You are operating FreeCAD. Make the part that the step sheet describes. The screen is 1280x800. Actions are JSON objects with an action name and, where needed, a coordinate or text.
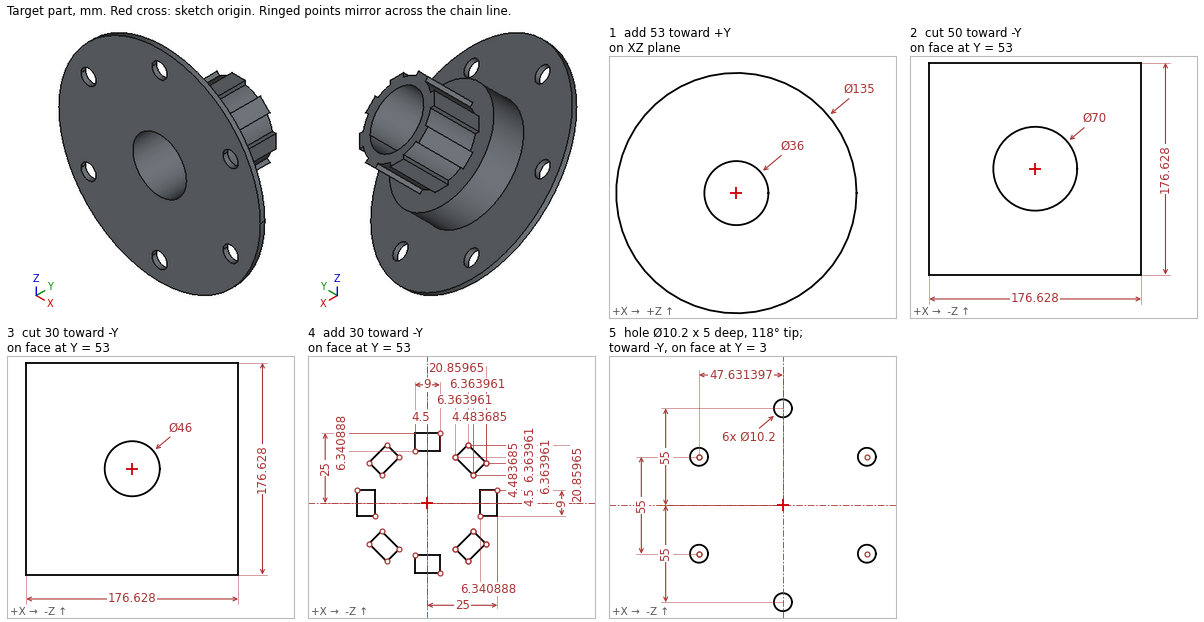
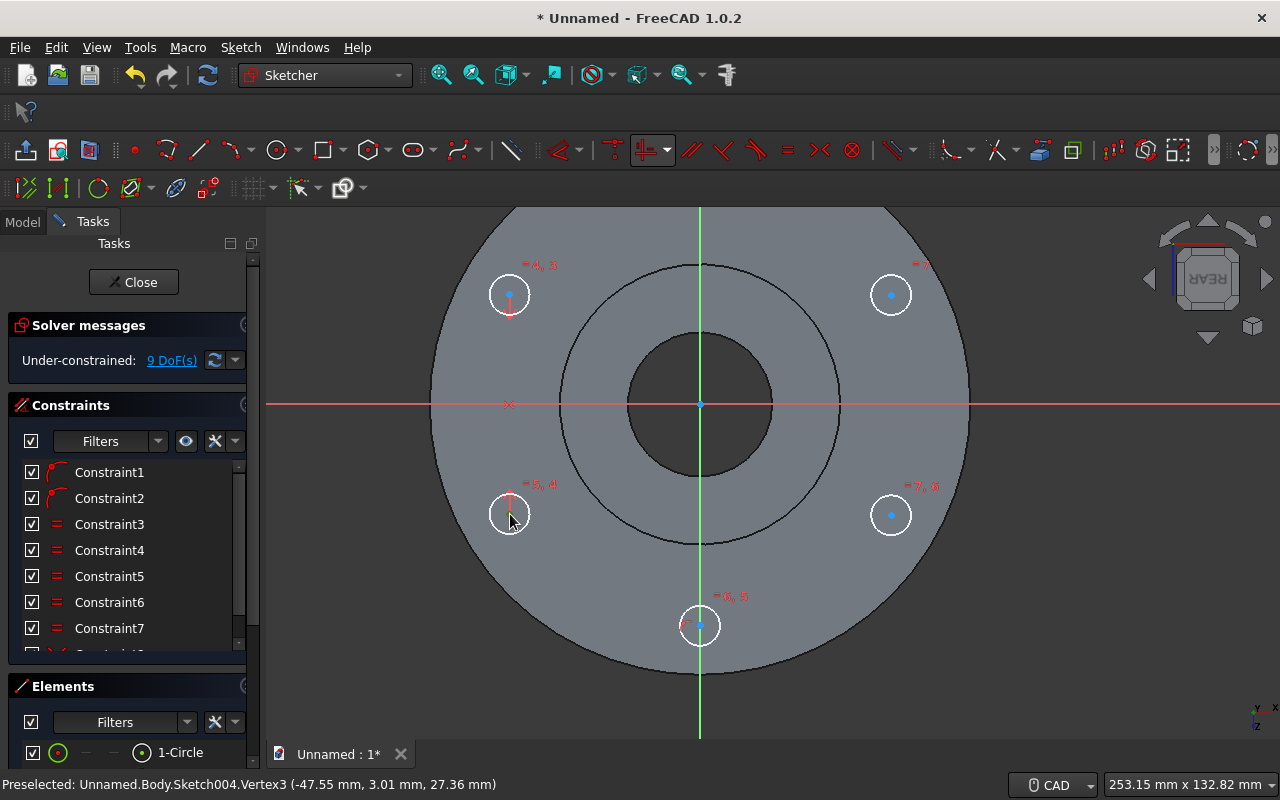
{"action": "left_click", "coordinate": [891, 515]}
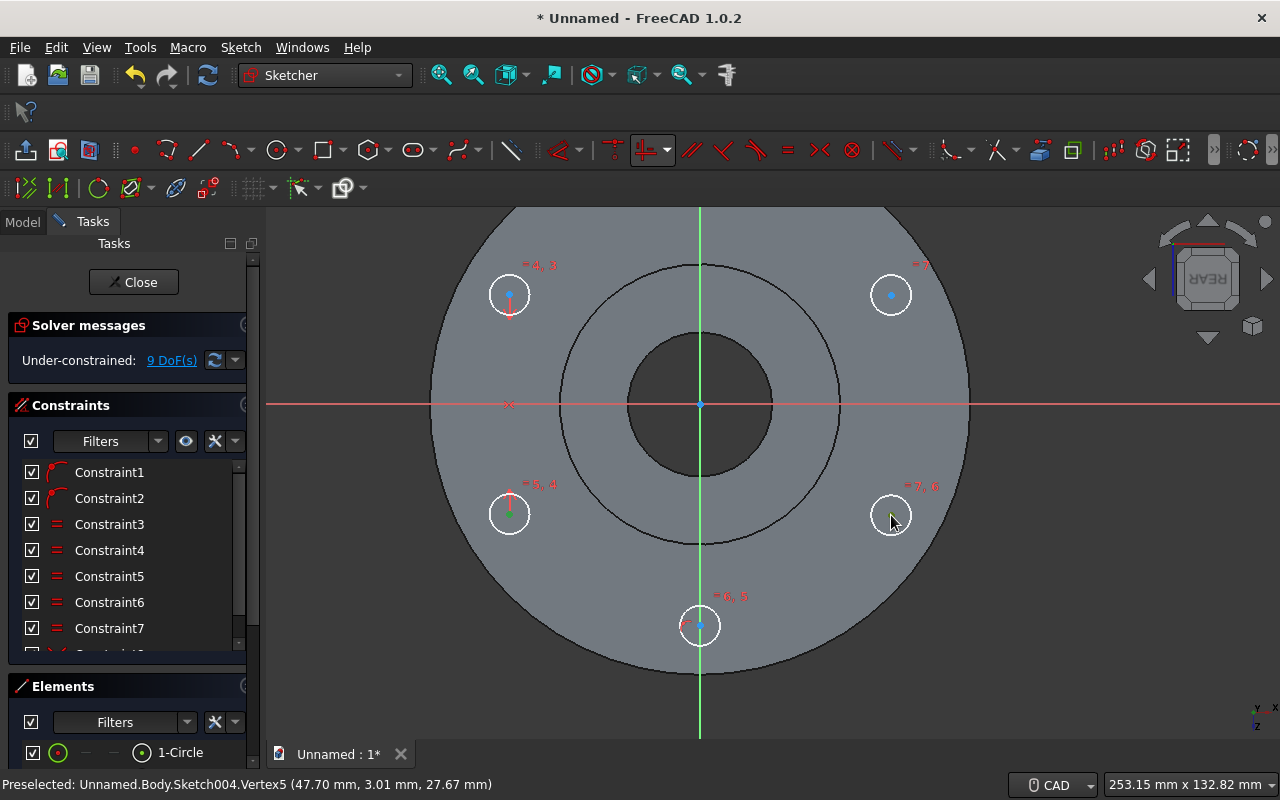
{"action": "left_click", "coordinate": [700, 677]}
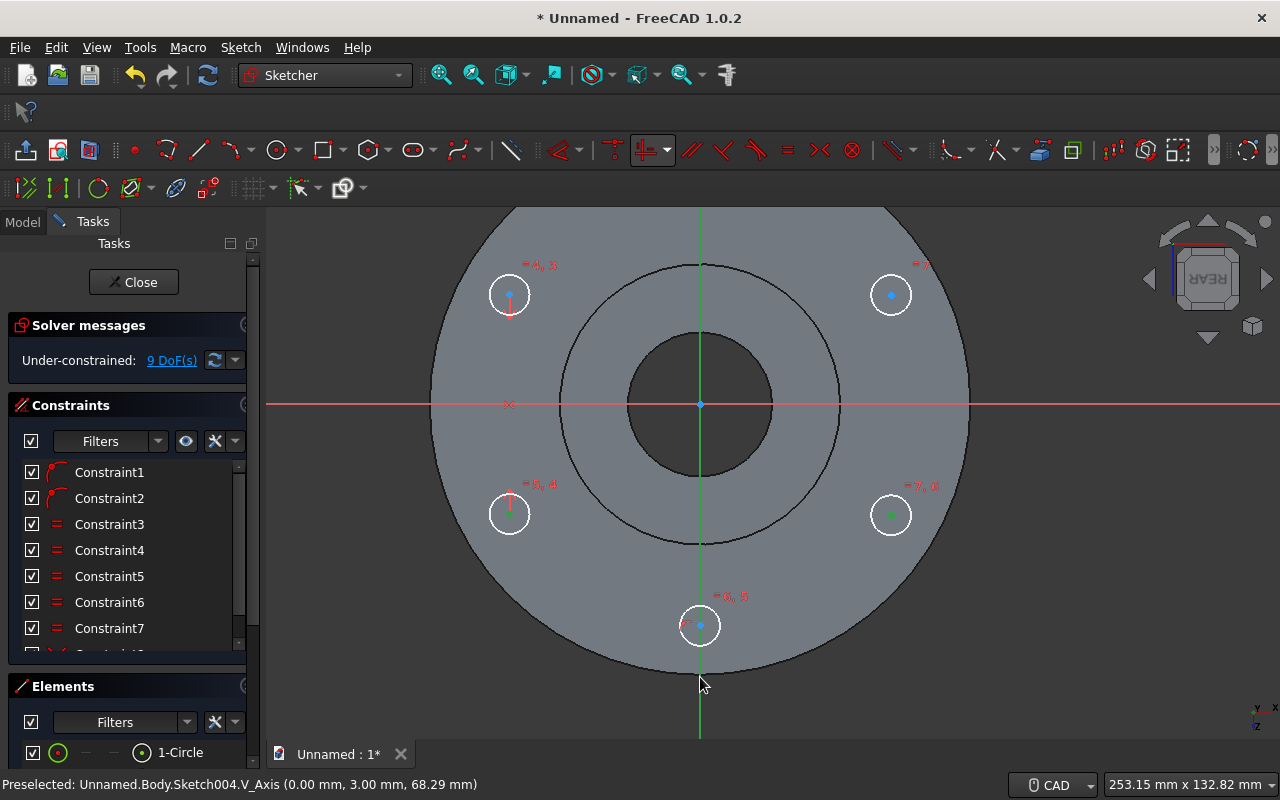
{"action": "left_click", "coordinate": [820, 150]}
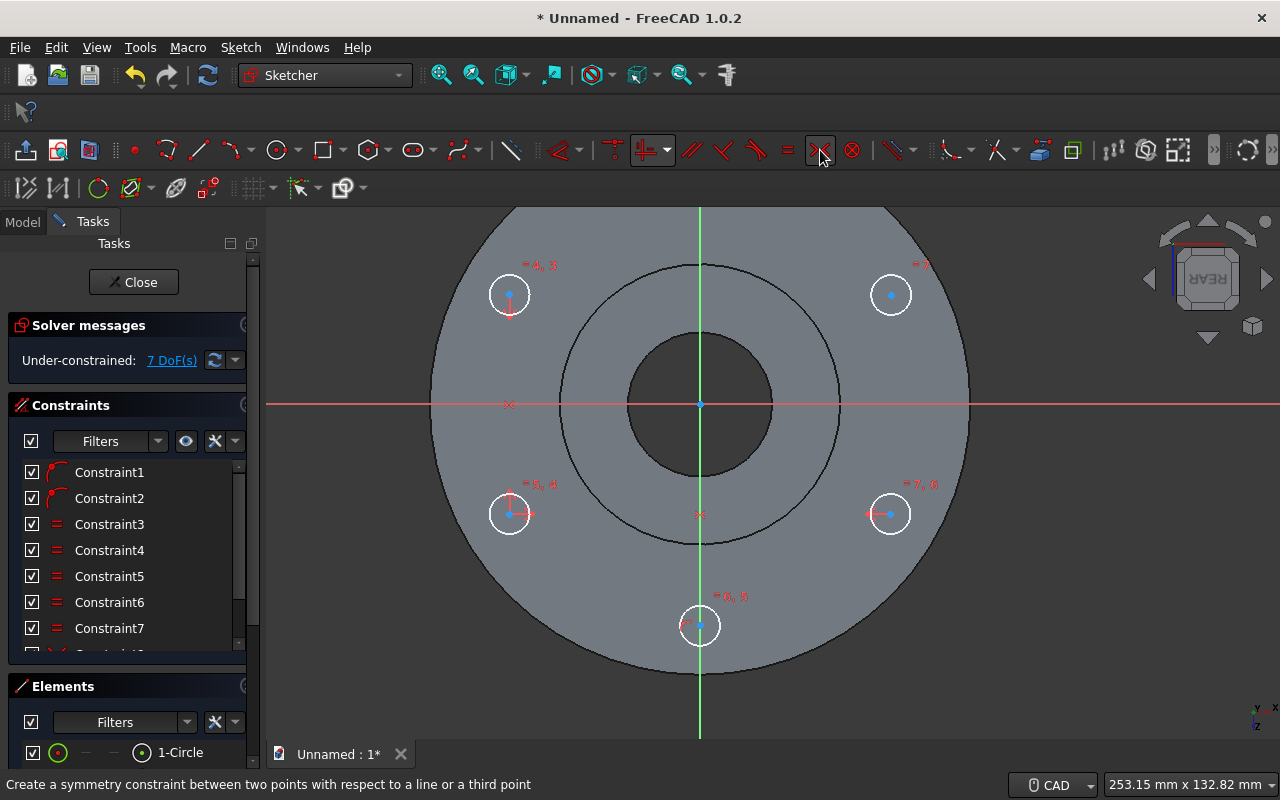
{"action": "left_click", "coordinate": [510, 295]}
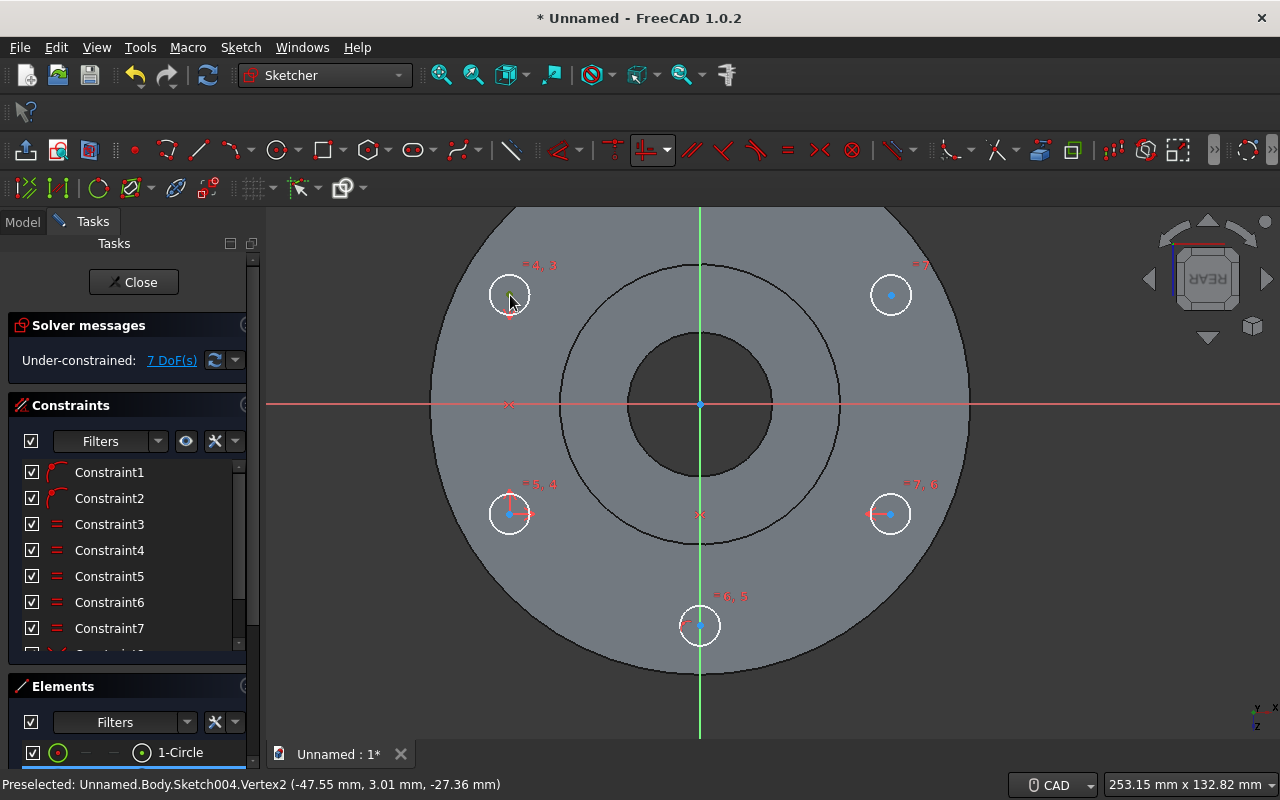
{"action": "left_click", "coordinate": [891, 295]}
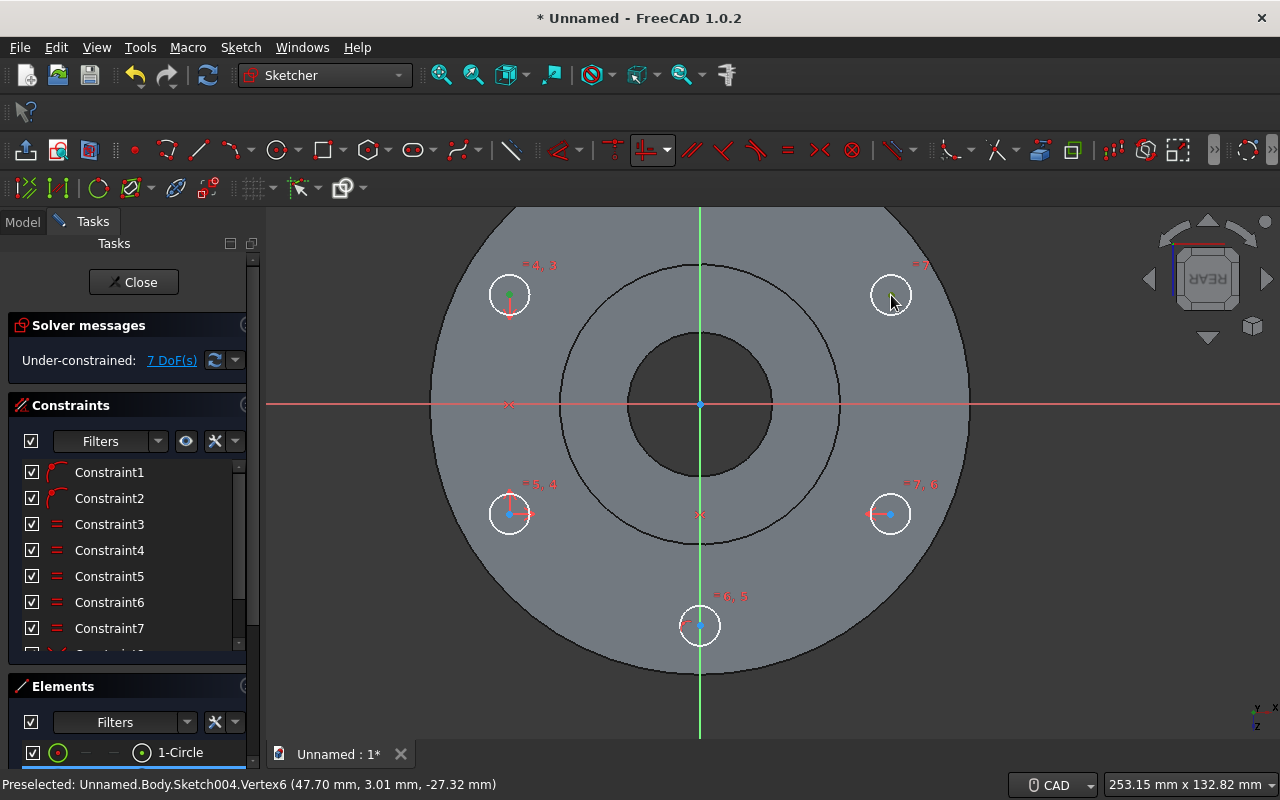
{"action": "left_click", "coordinate": [700, 677]}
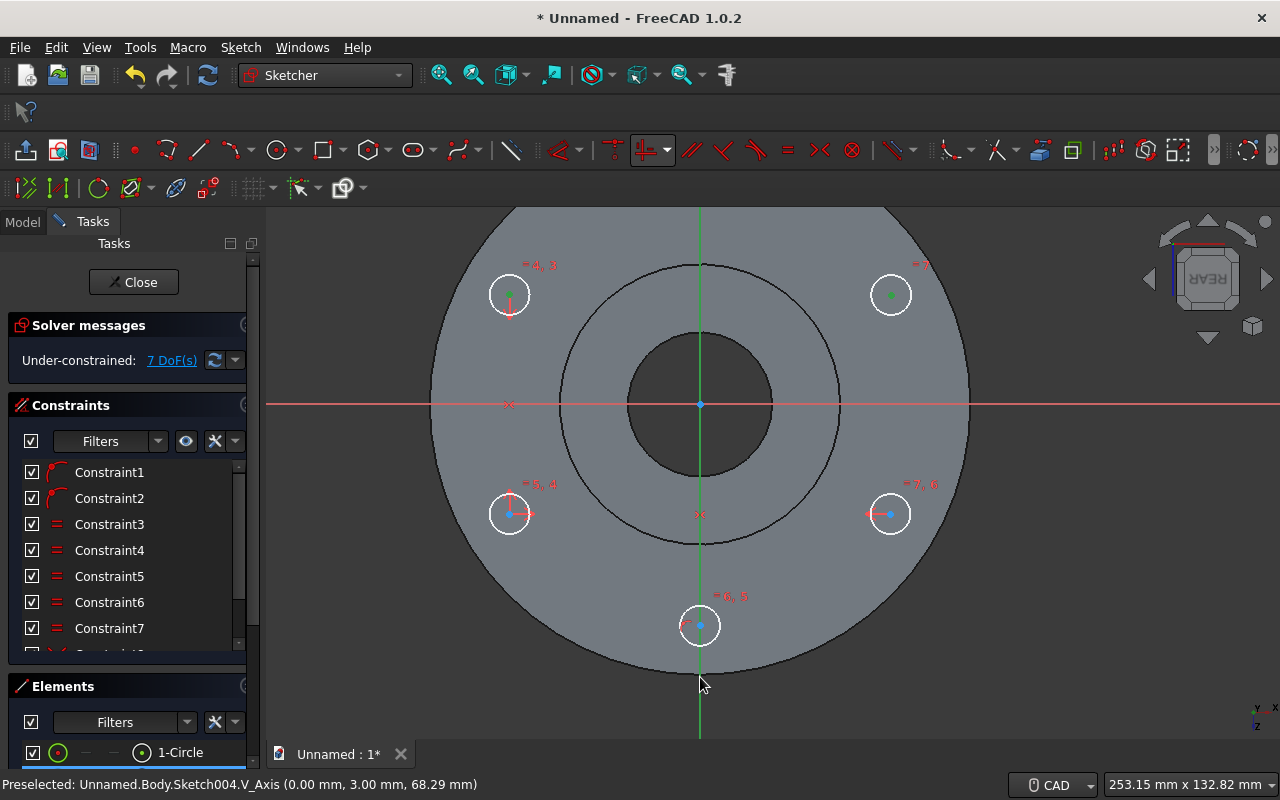
{"action": "left_click", "coordinate": [820, 150]}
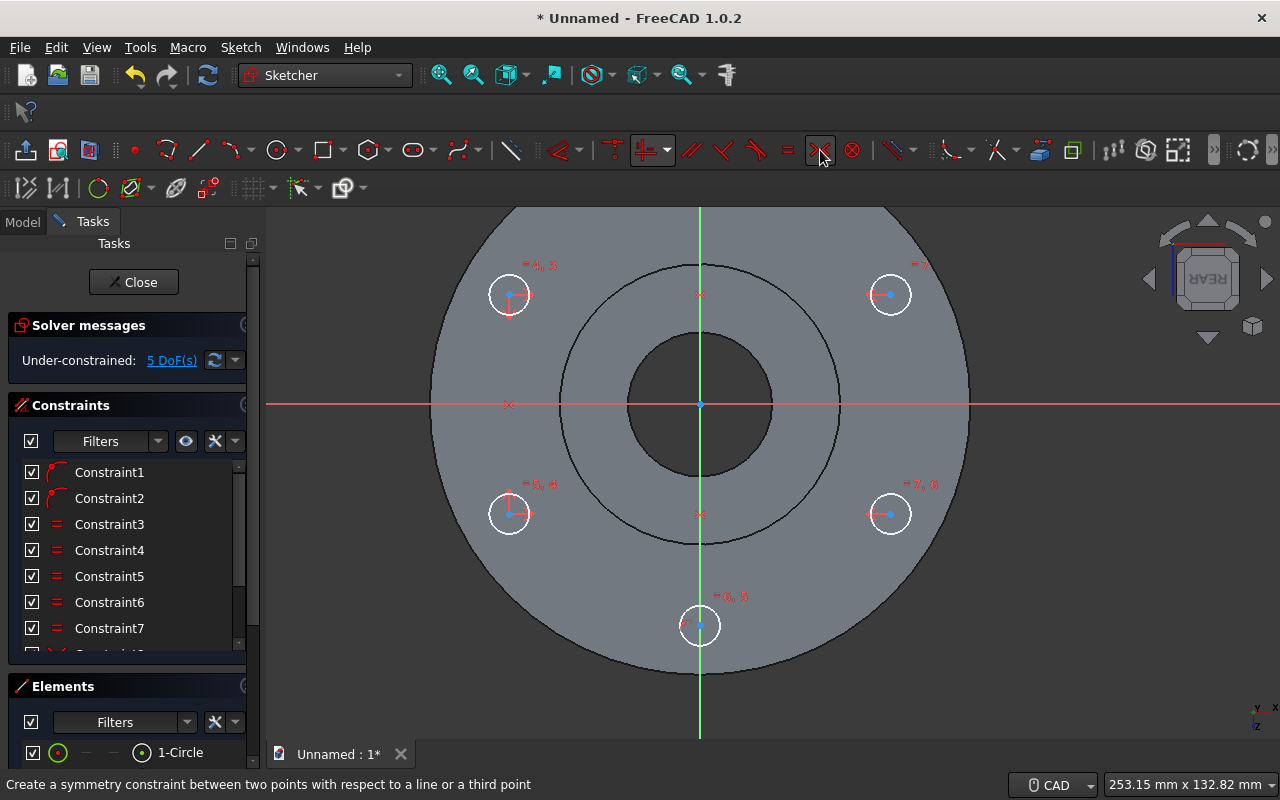
{"action": "left_click", "coordinate": [558, 150]}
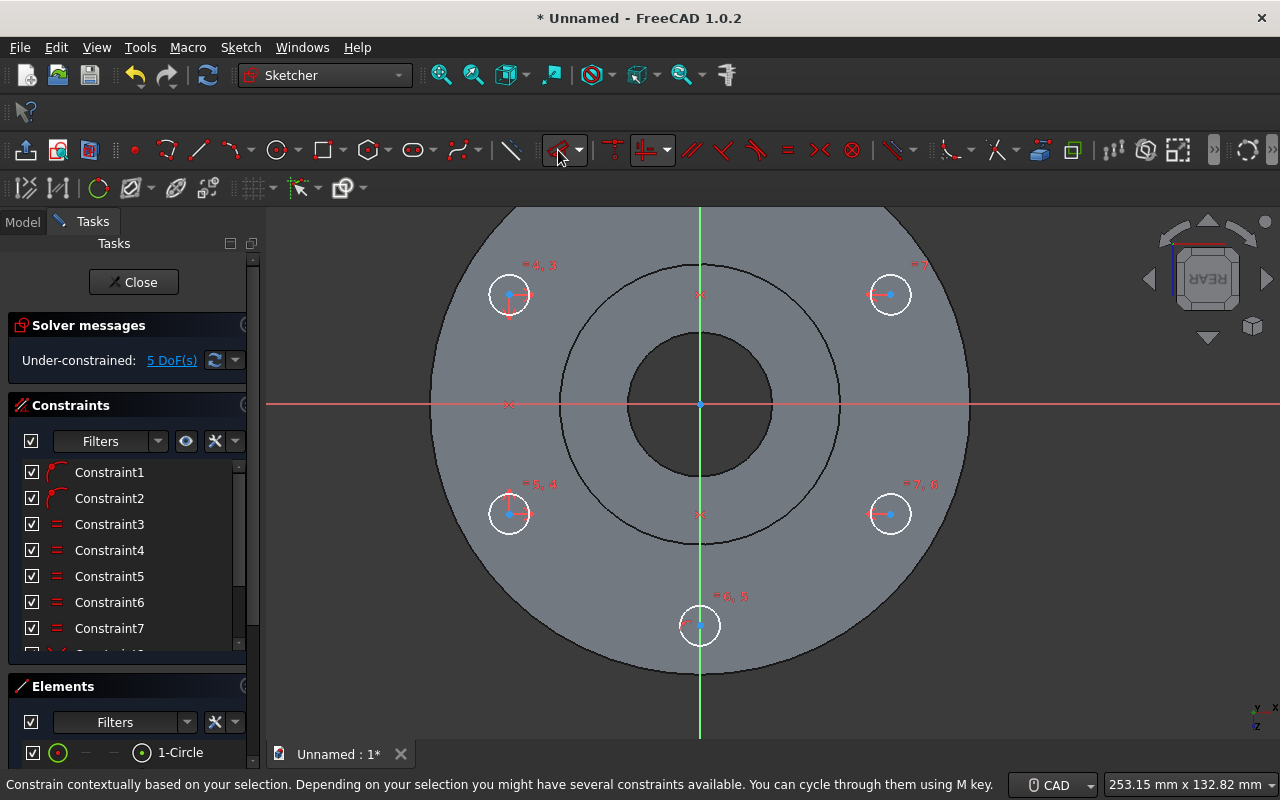
{"action": "scroll", "coordinate": [714, 612], "scroll_direction": "down", "scroll_amount": 2}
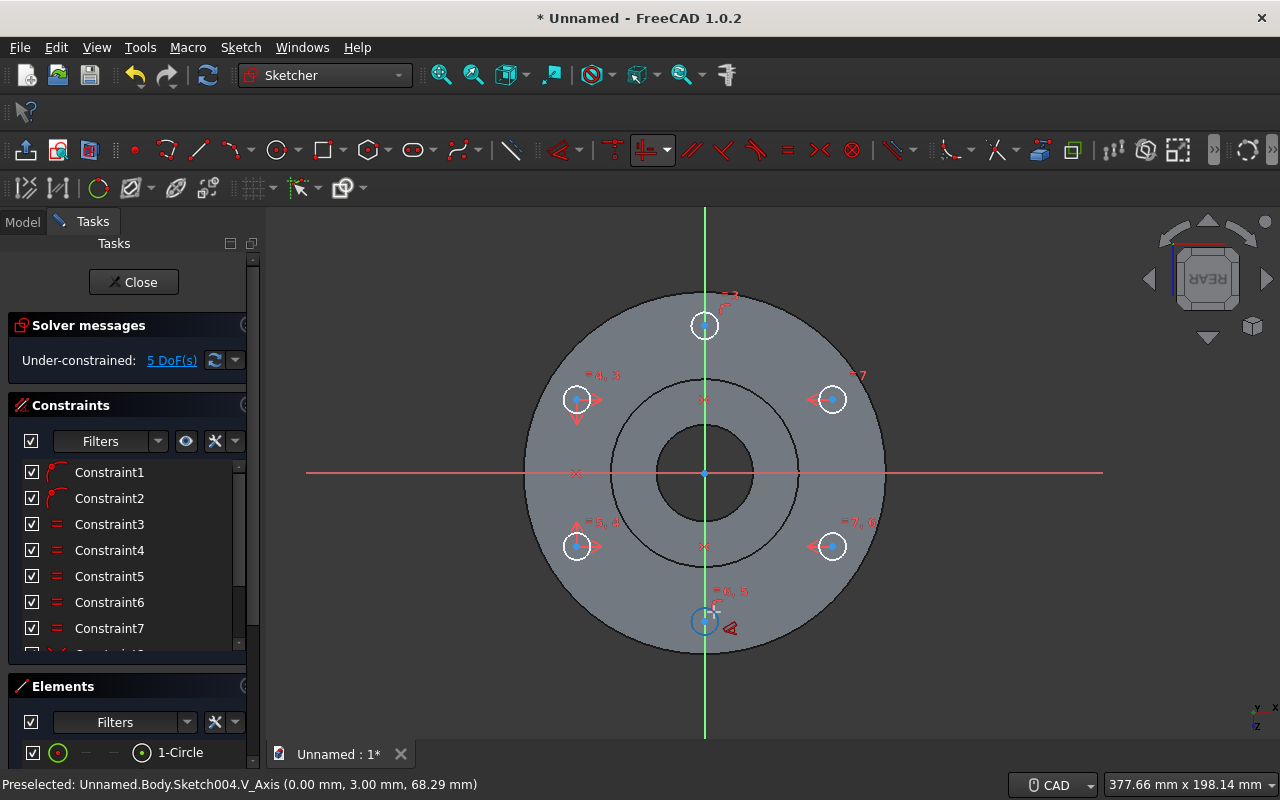
{"action": "scroll", "coordinate": [714, 316], "scroll_direction": "up", "scroll_amount": 2}